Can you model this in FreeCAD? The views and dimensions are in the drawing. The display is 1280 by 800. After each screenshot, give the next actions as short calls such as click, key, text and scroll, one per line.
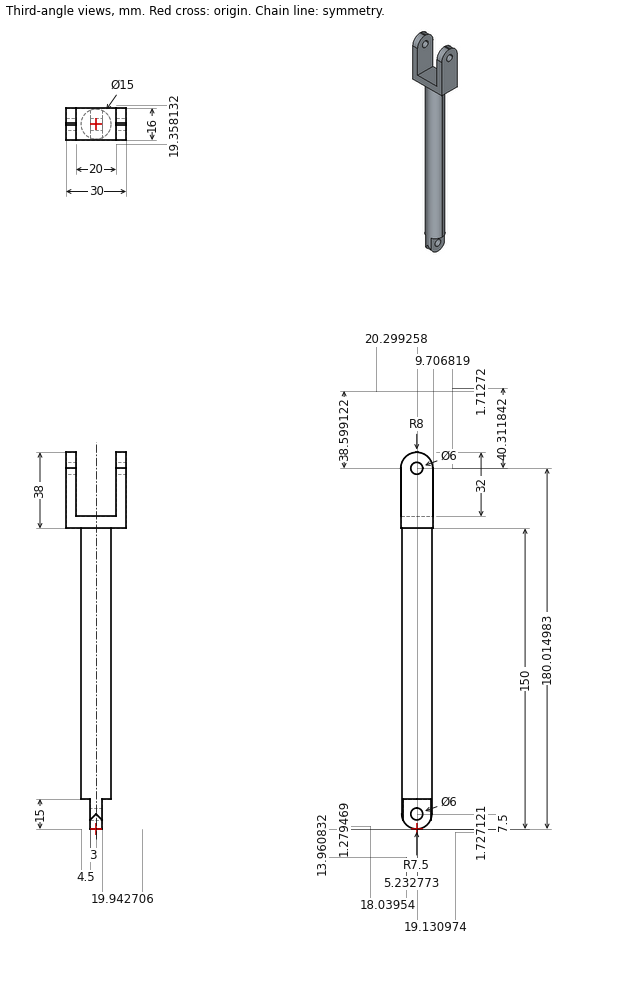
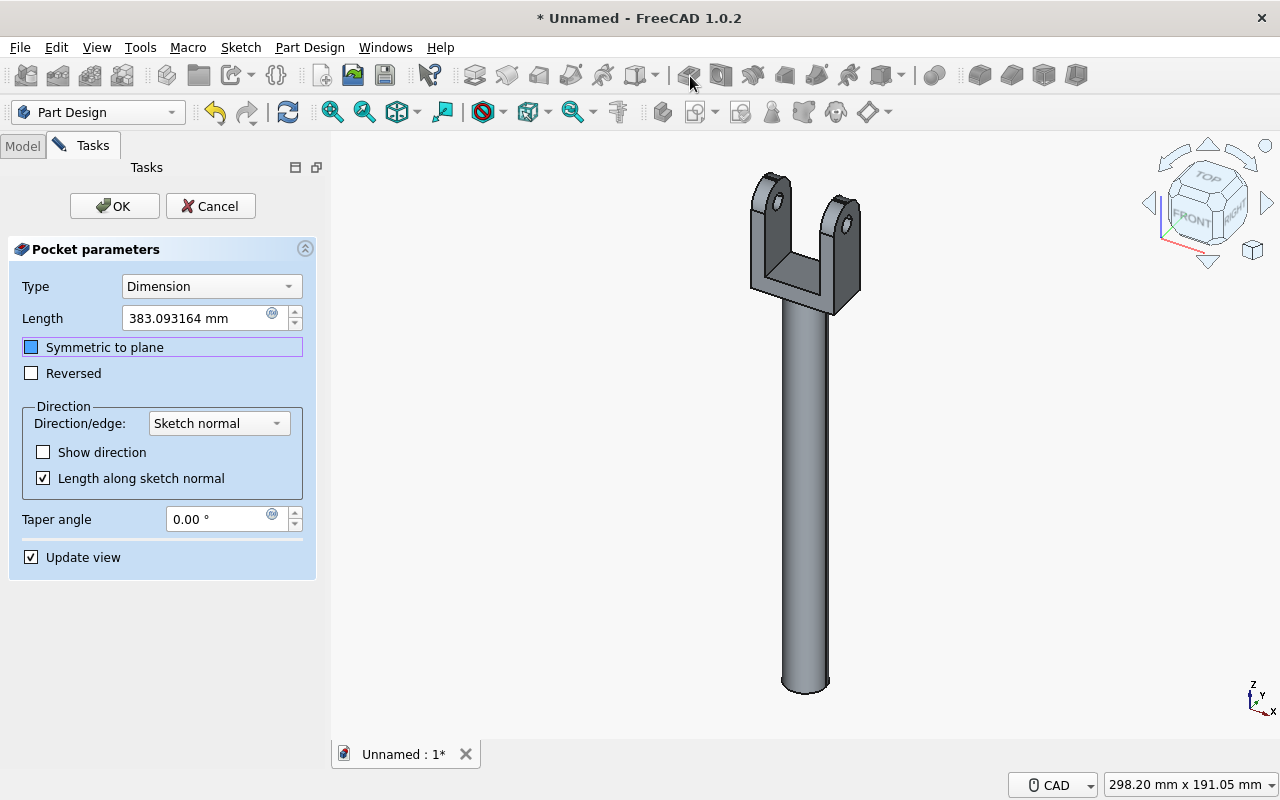
click(30, 347)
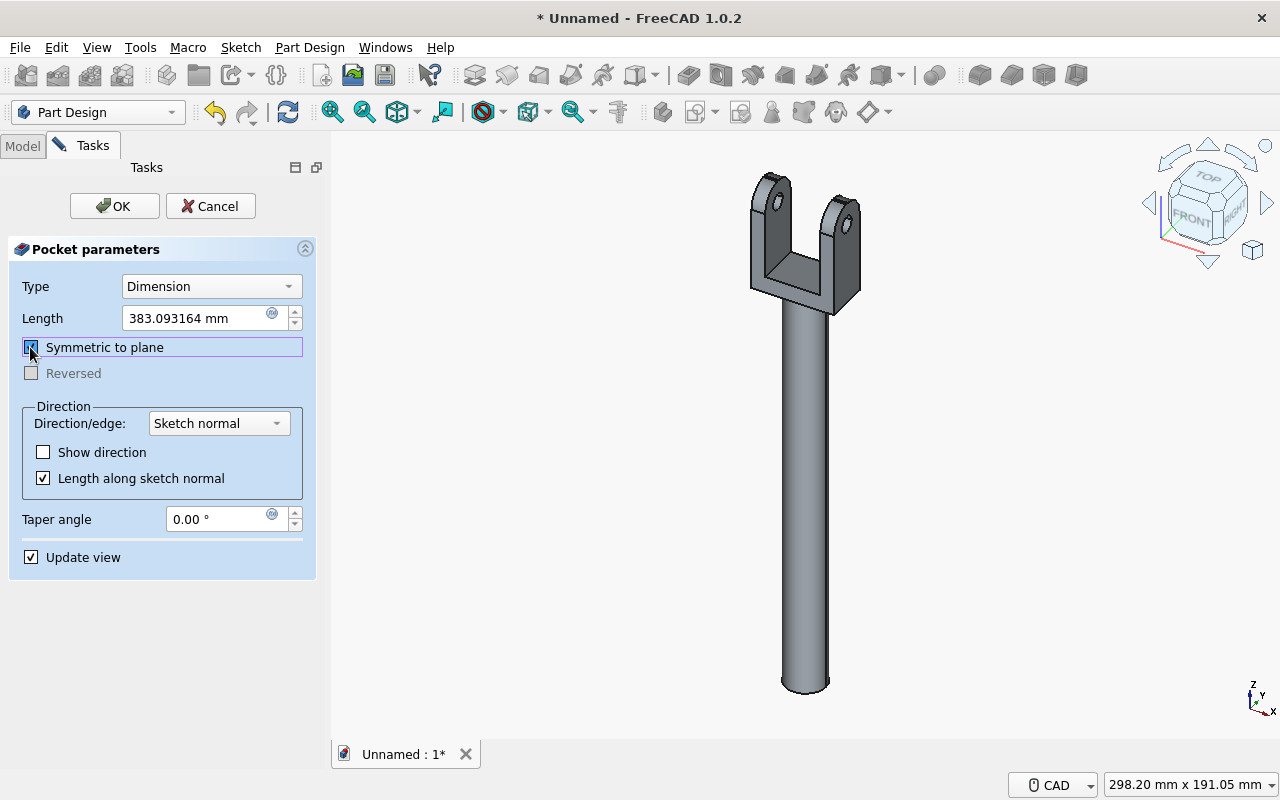
click(115, 206)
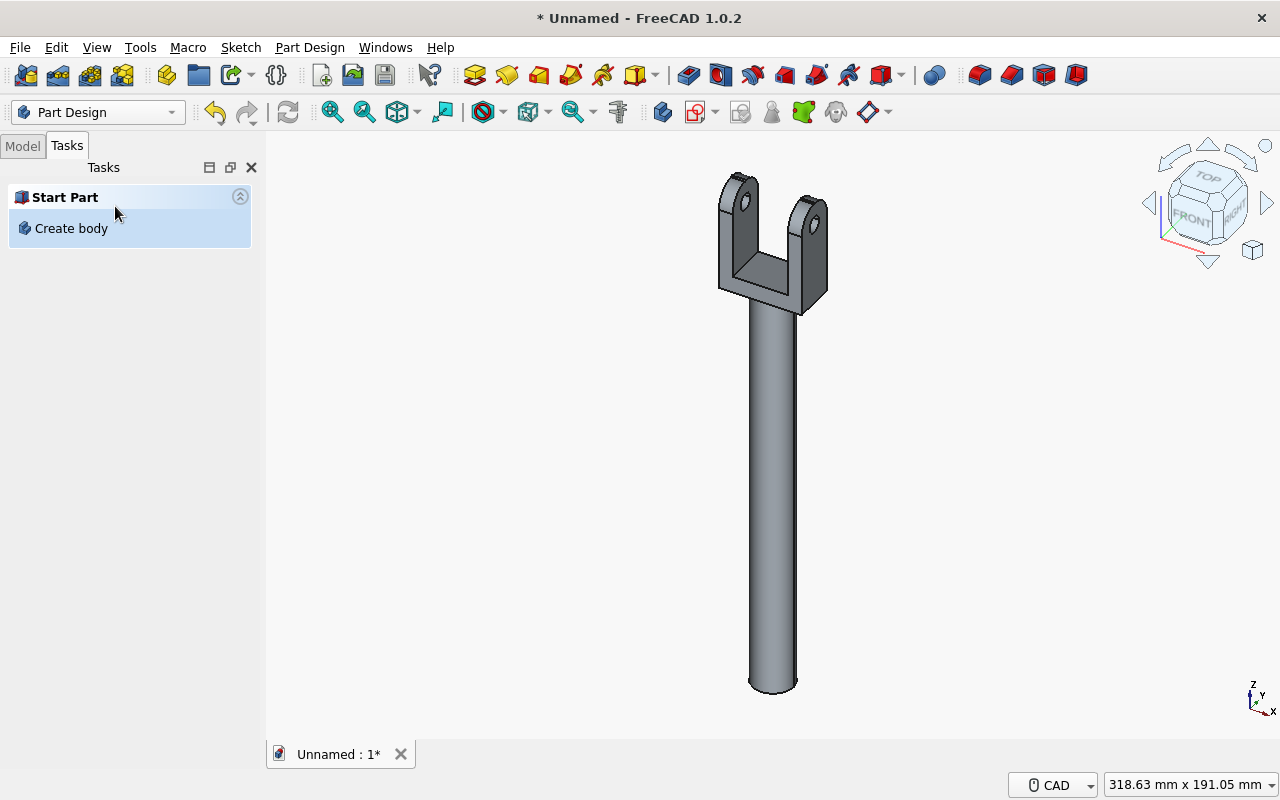
click(696, 112)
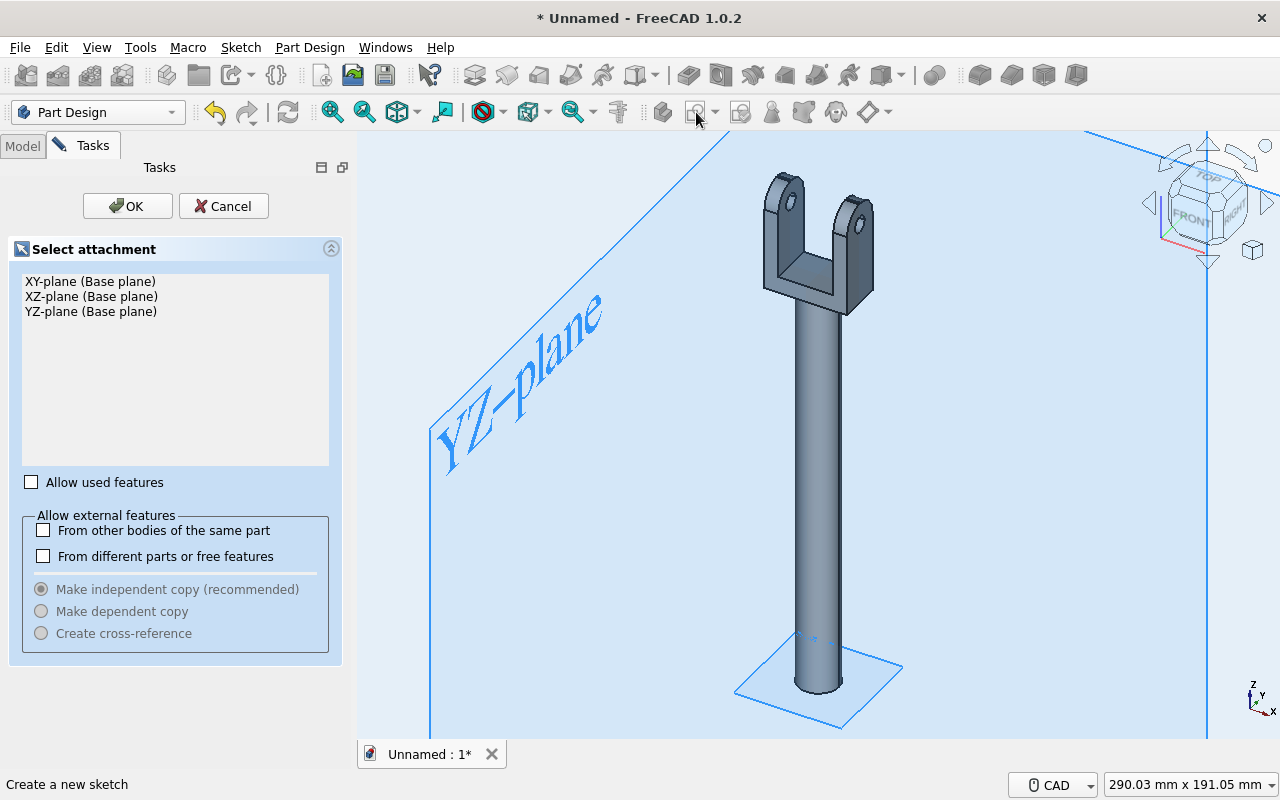
click(82, 296)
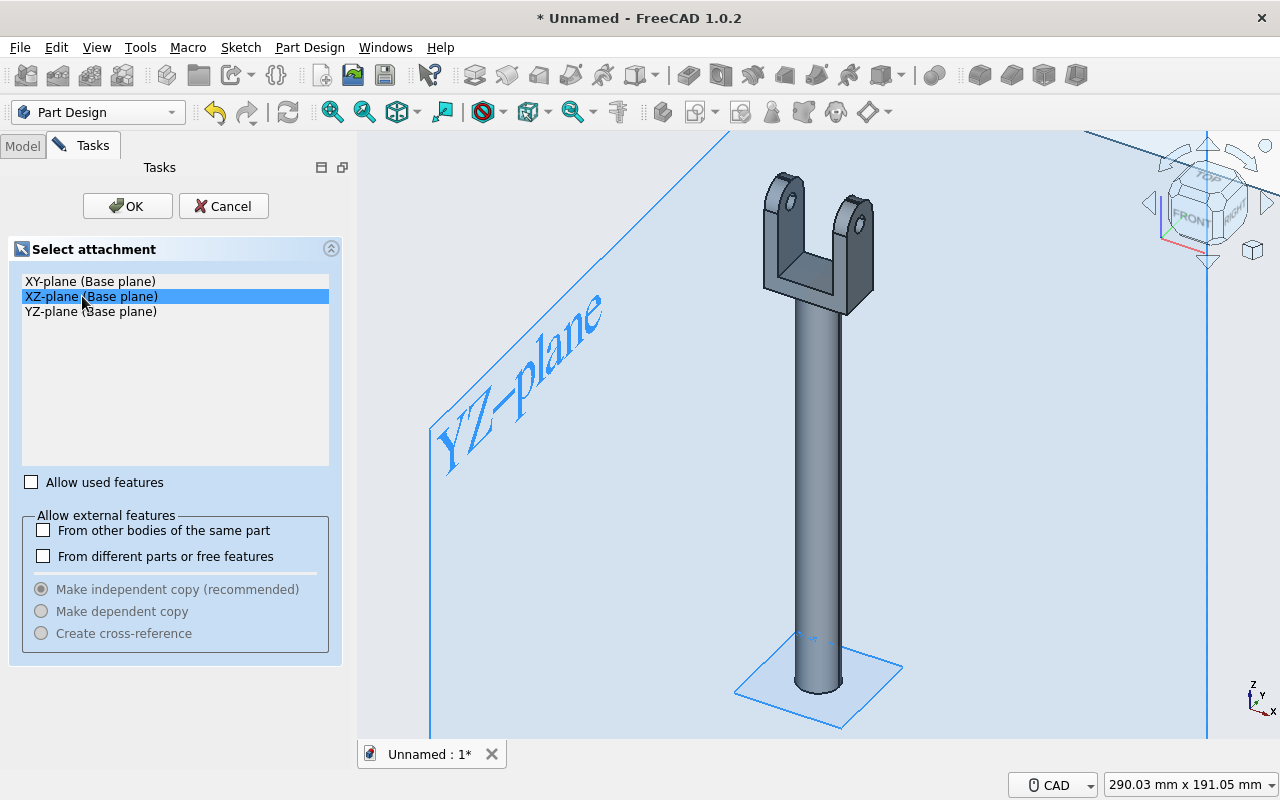
click(128, 206)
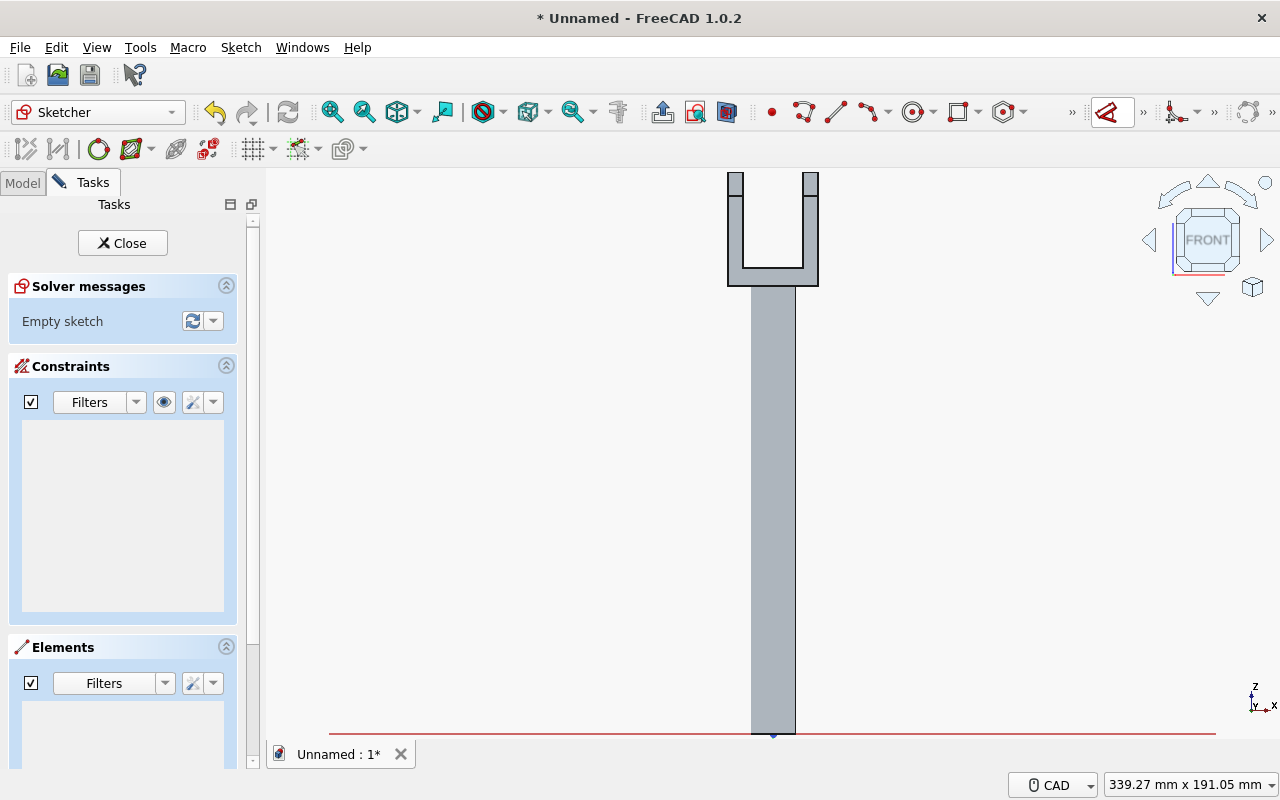
key(q)
key(s)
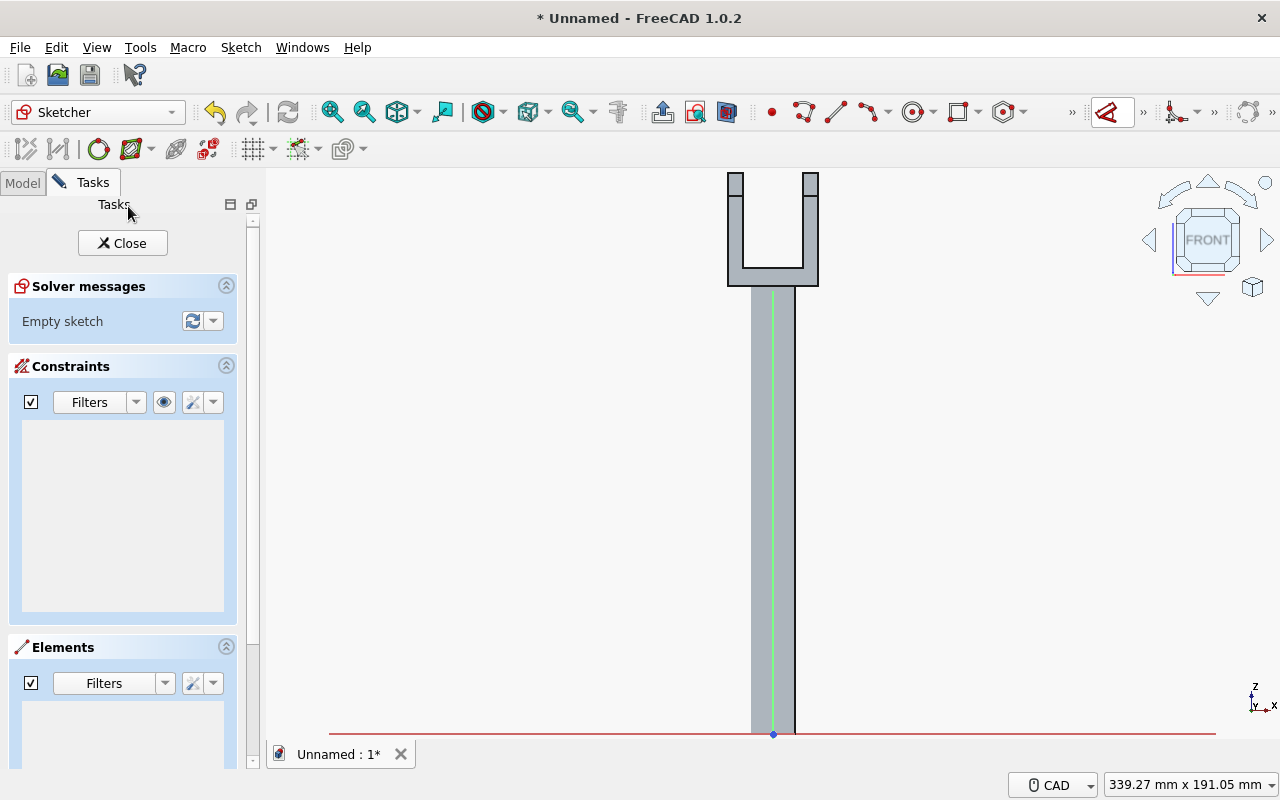
scroll(704, 454, down, 5)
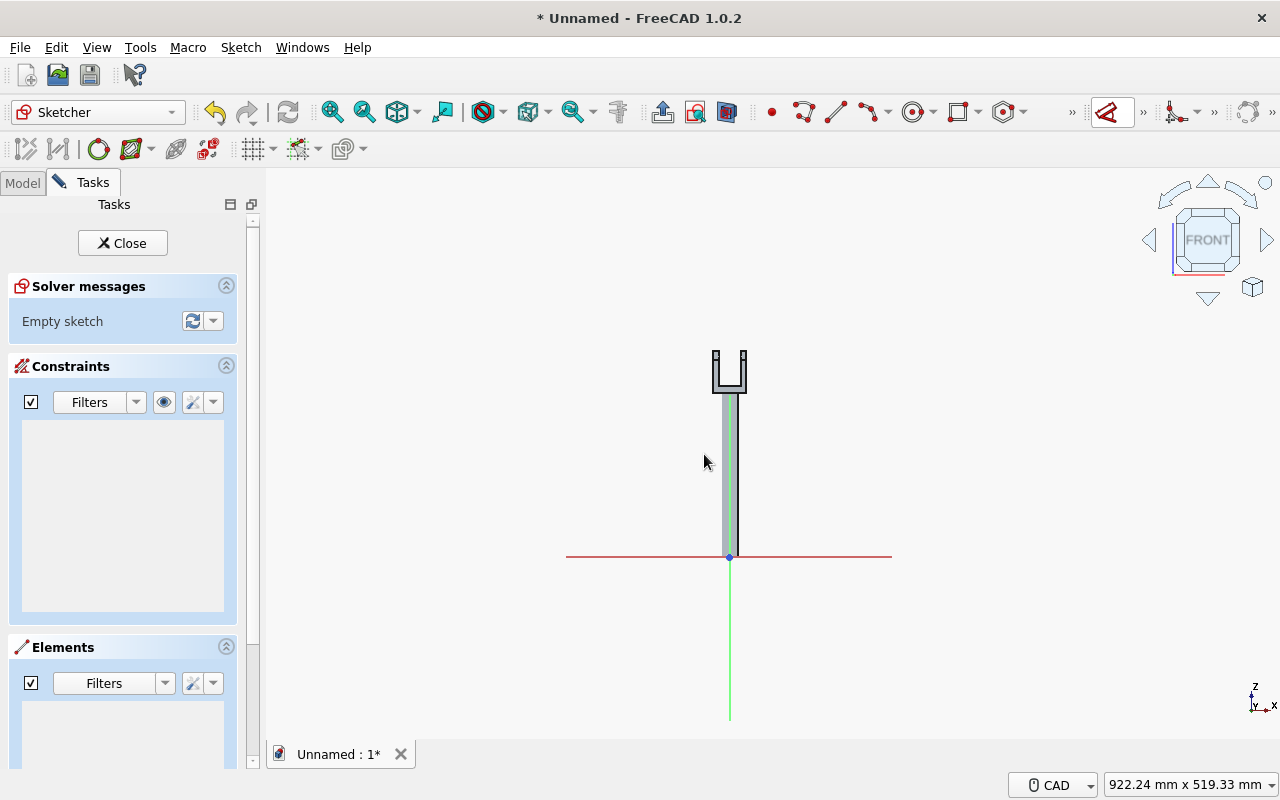
scroll(740, 555, up, 14)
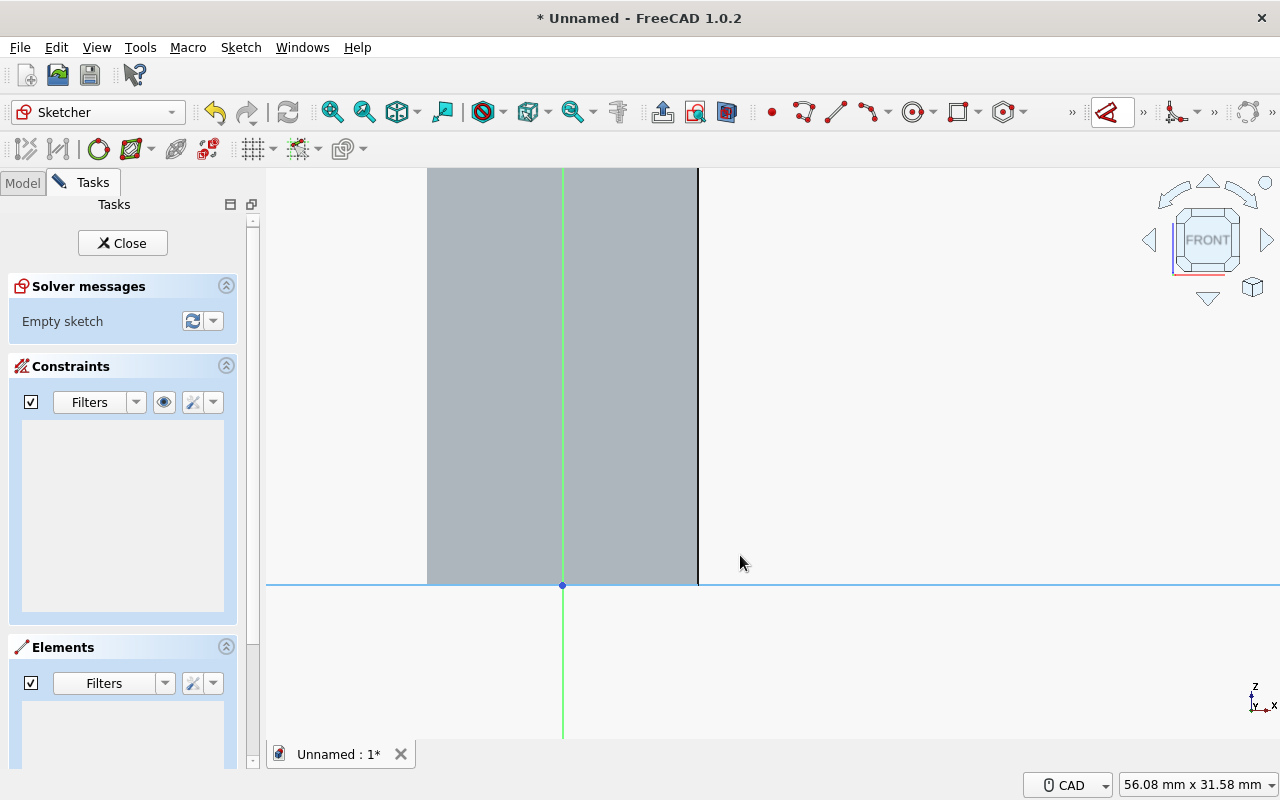
click(958, 112)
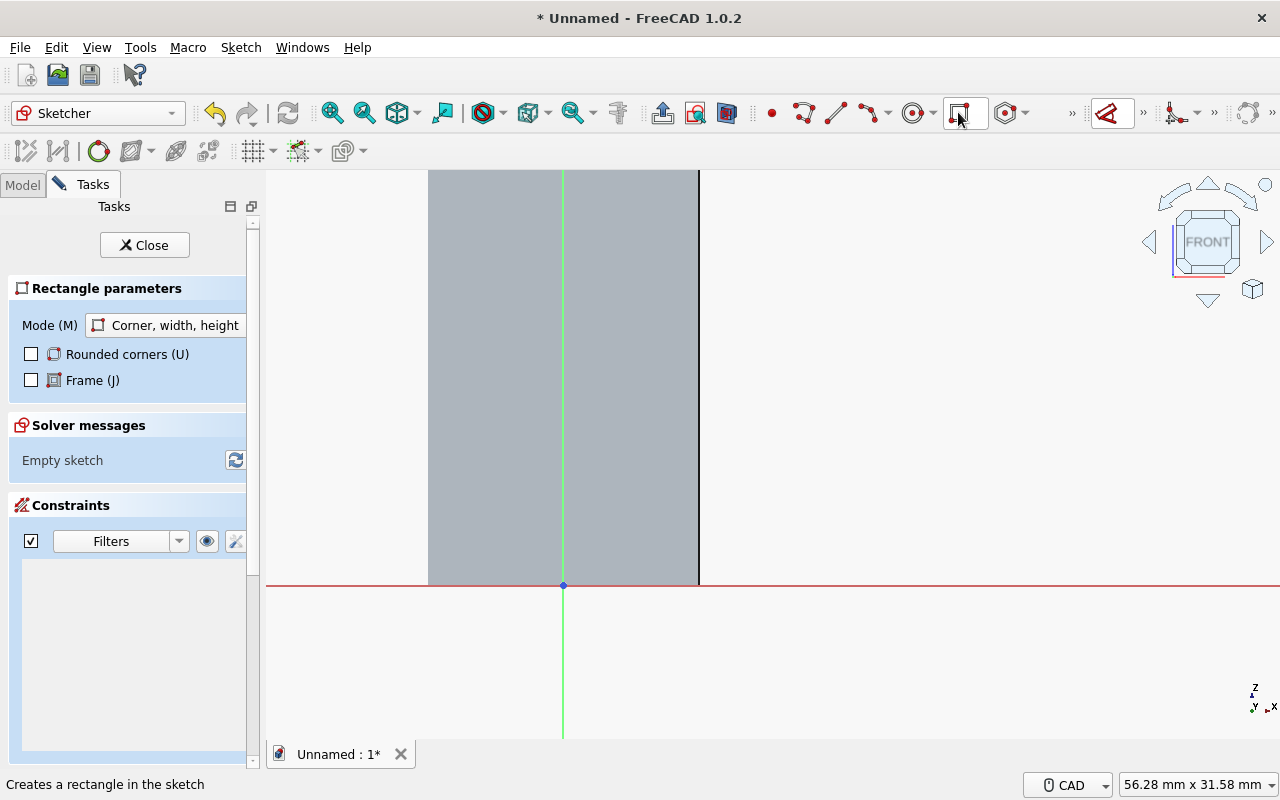
click(428, 316)
click(509, 586)